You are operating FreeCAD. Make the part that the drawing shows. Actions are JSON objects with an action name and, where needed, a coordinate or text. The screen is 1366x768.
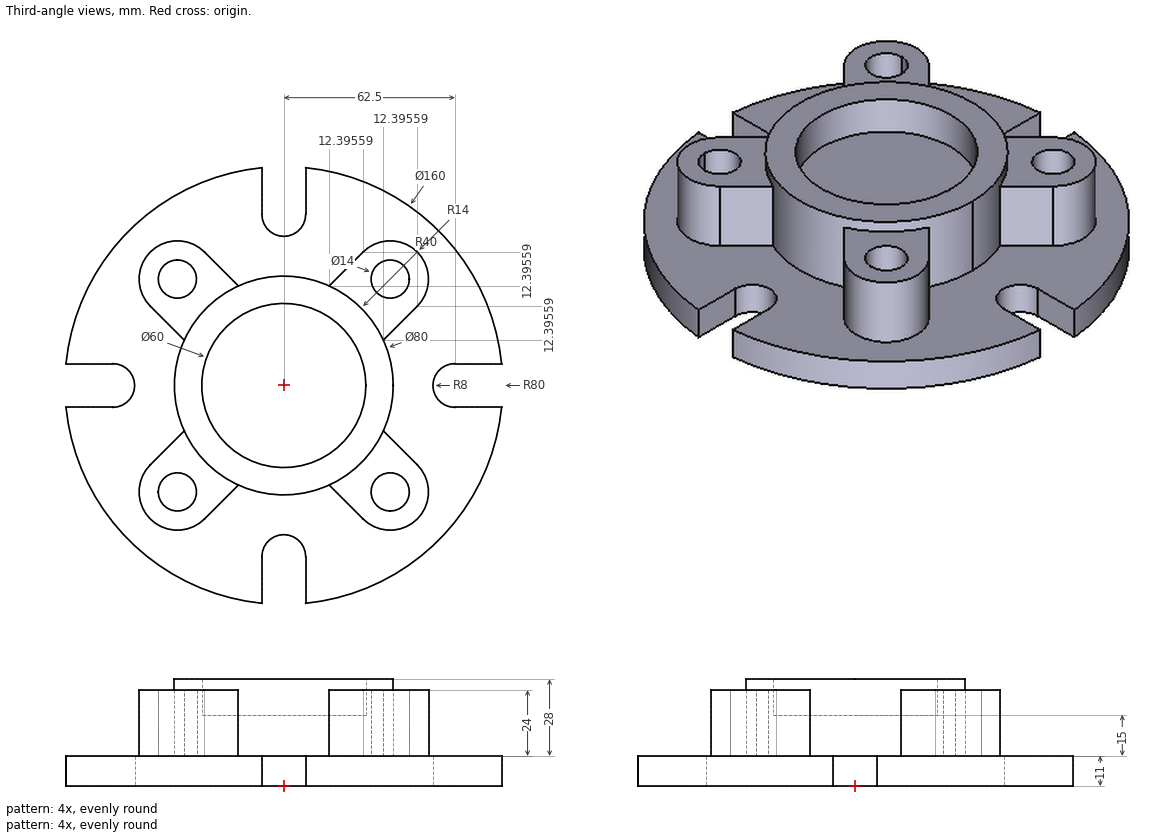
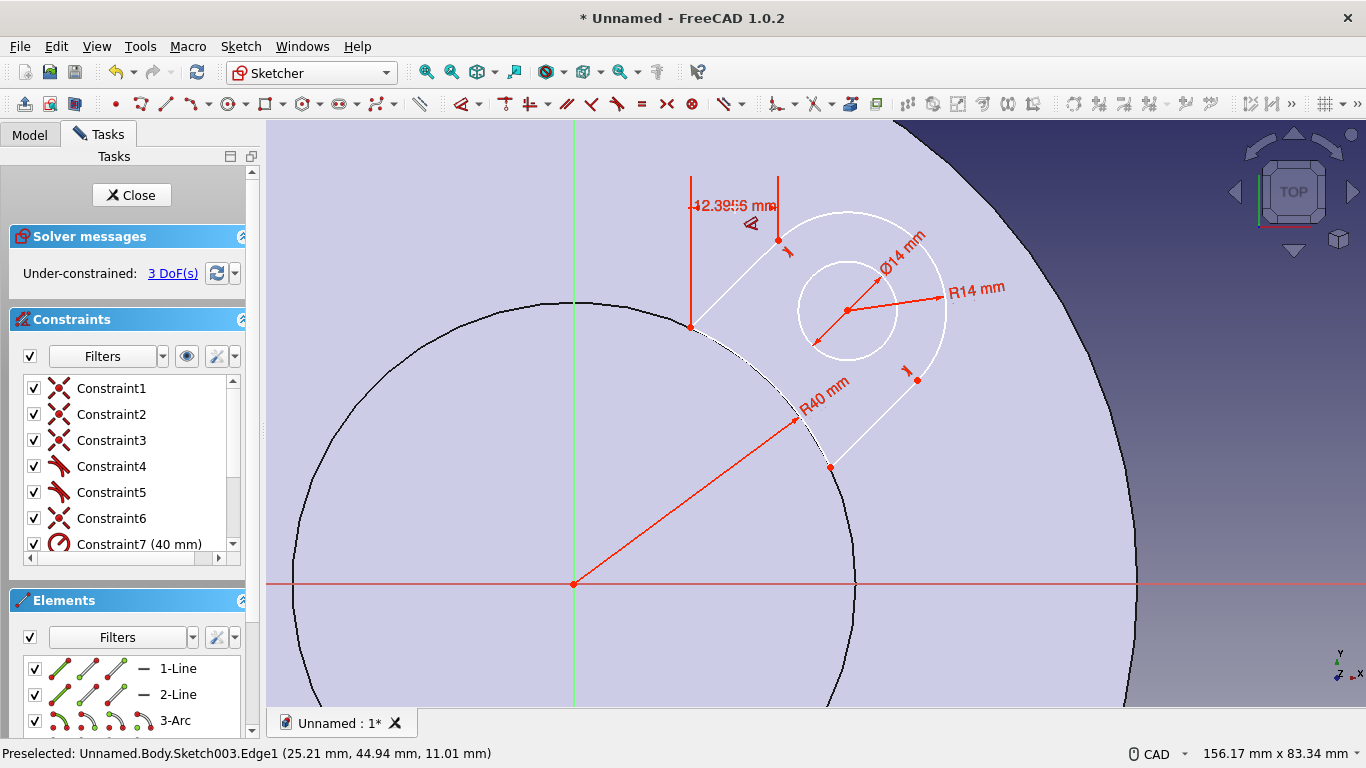
{"action": "left_click", "coordinate": [752, 267]}
{"action": "left_click", "coordinate": [657, 284]}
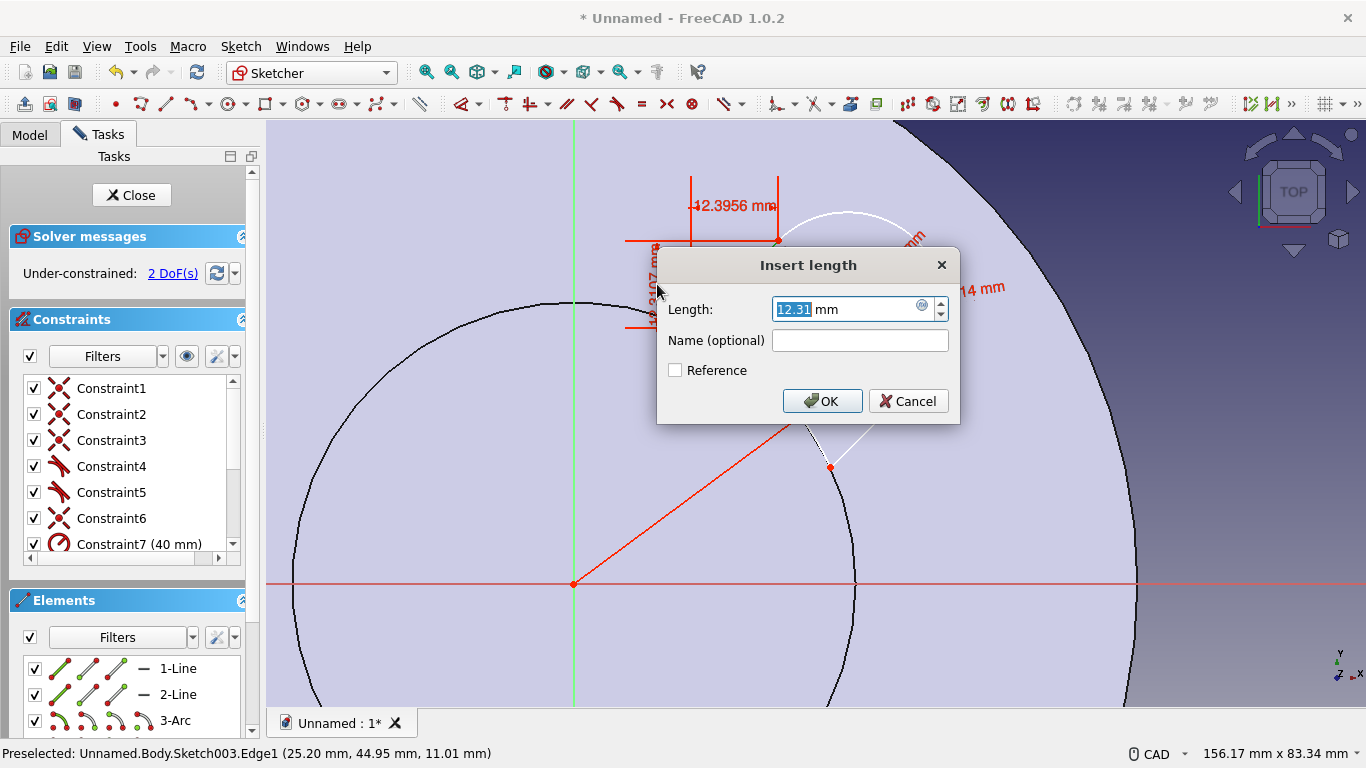
{"action": "type", "text": "12.39559"}
{"action": "key", "text": "Return"}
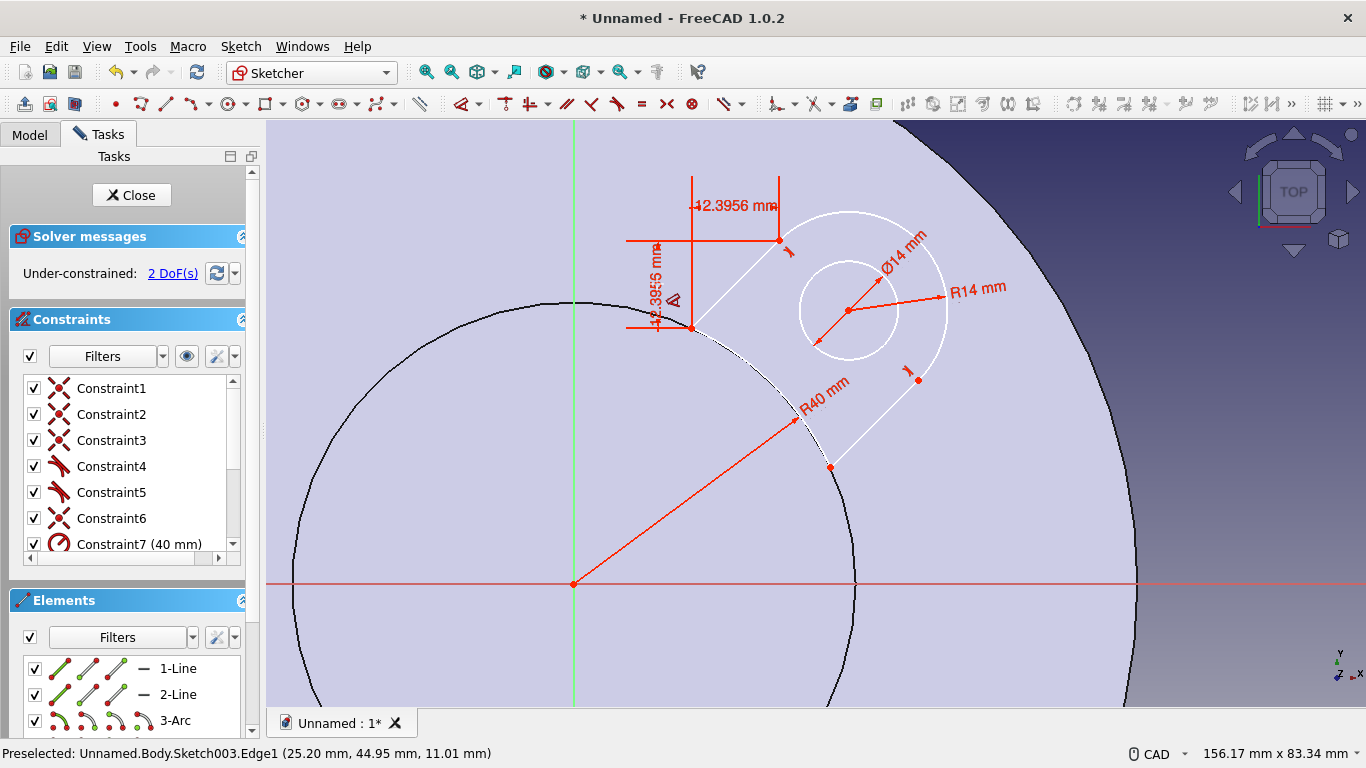
{"action": "left_click", "coordinate": [857, 442]}
{"action": "left_click", "coordinate": [875, 502]}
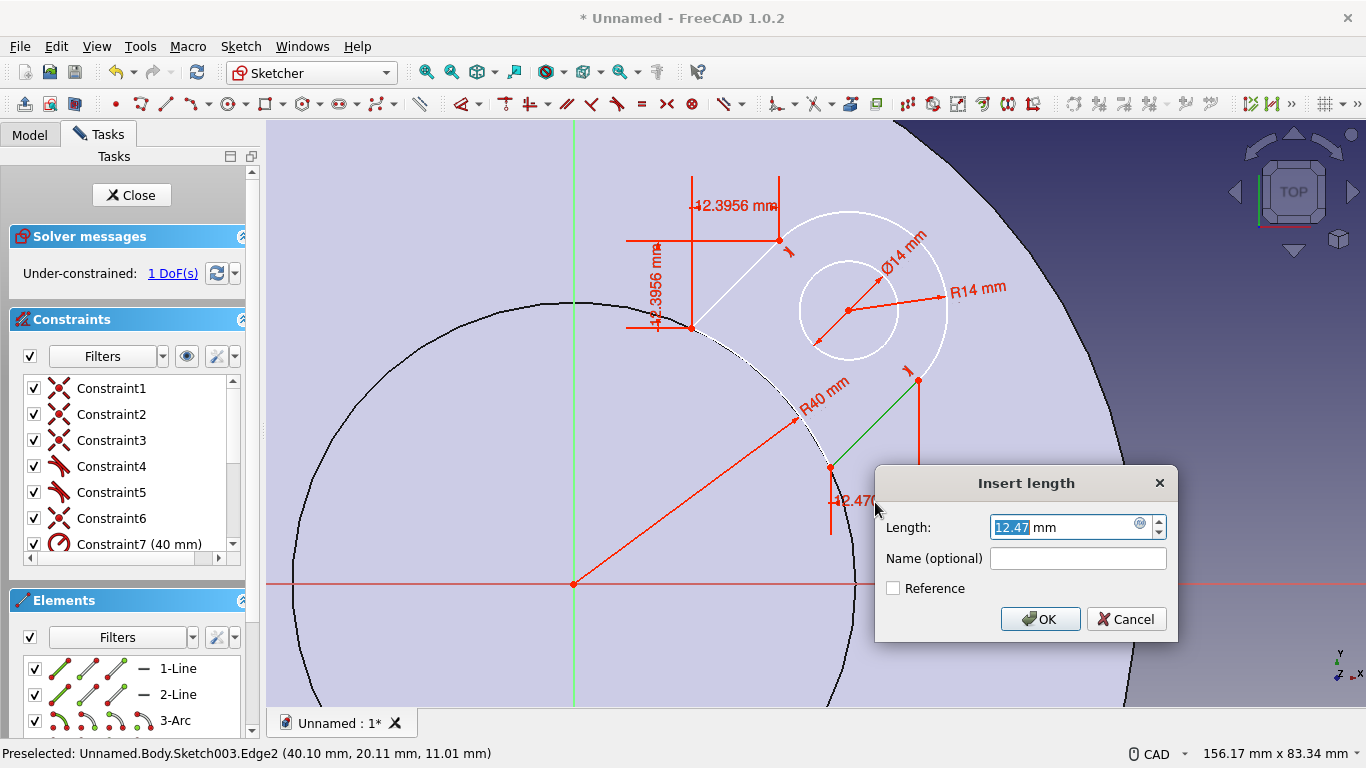
{"action": "type", "text": "12.39559"}
{"action": "key", "text": "Return"}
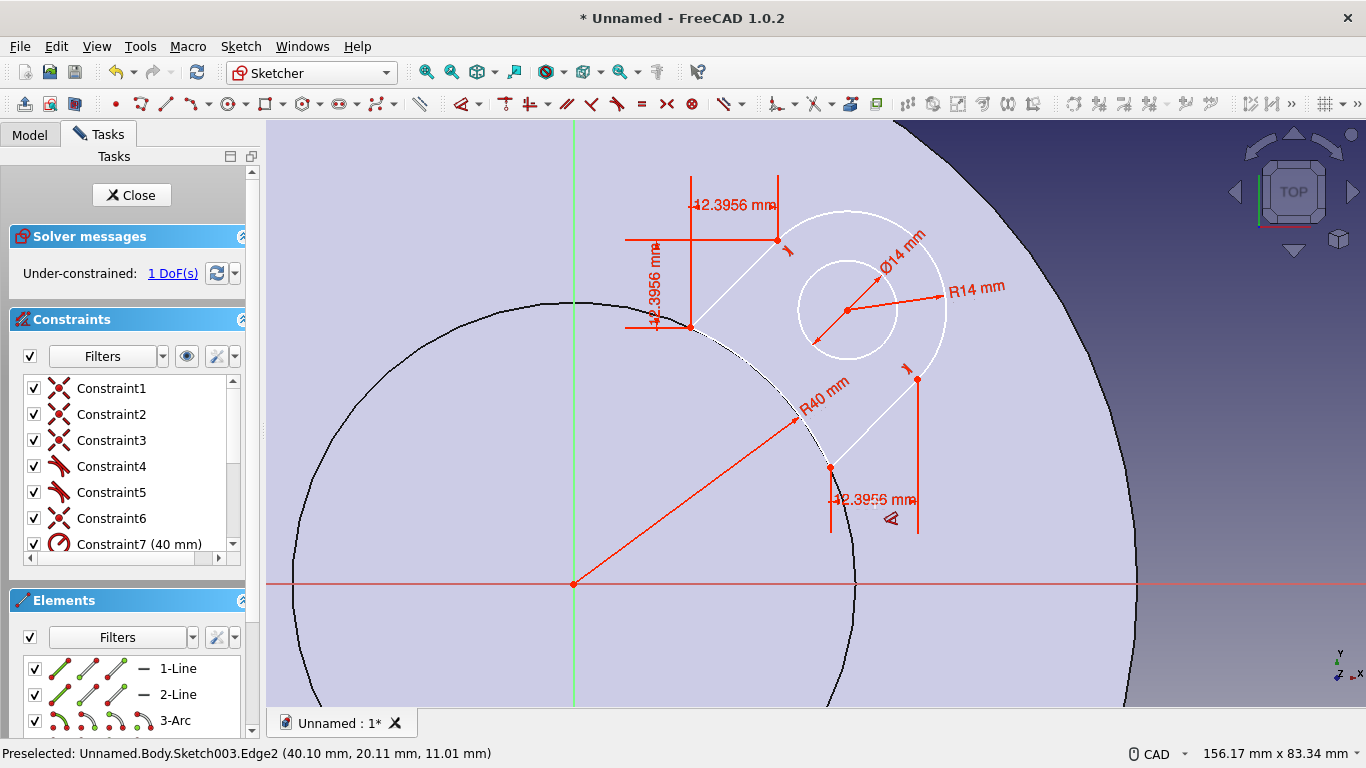
{"action": "left_click", "coordinate": [857, 441]}
{"action": "left_click", "coordinate": [952, 424]}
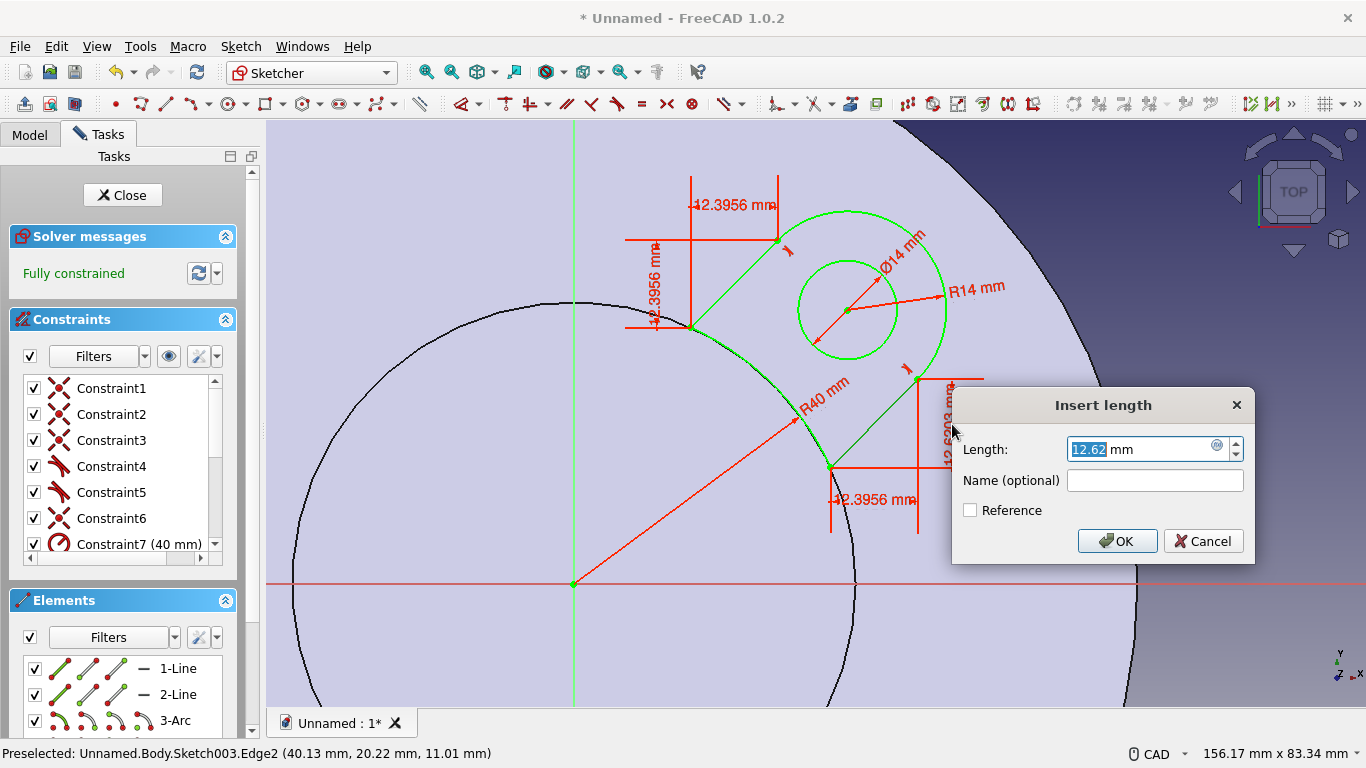
{"action": "type", "text": "12.39559"}
{"action": "key", "text": "Return"}
{"action": "key", "text": "Escape"}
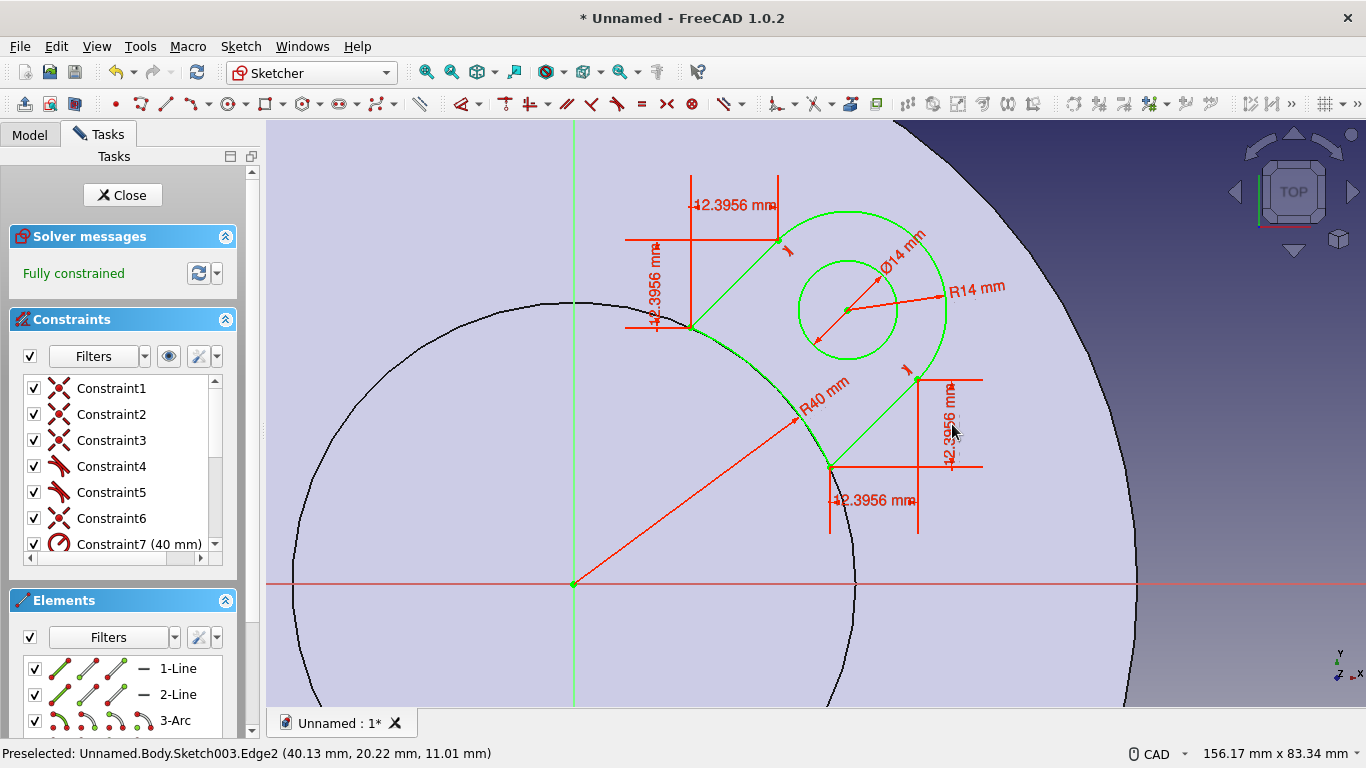
{"action": "left_click", "coordinate": [123, 195]}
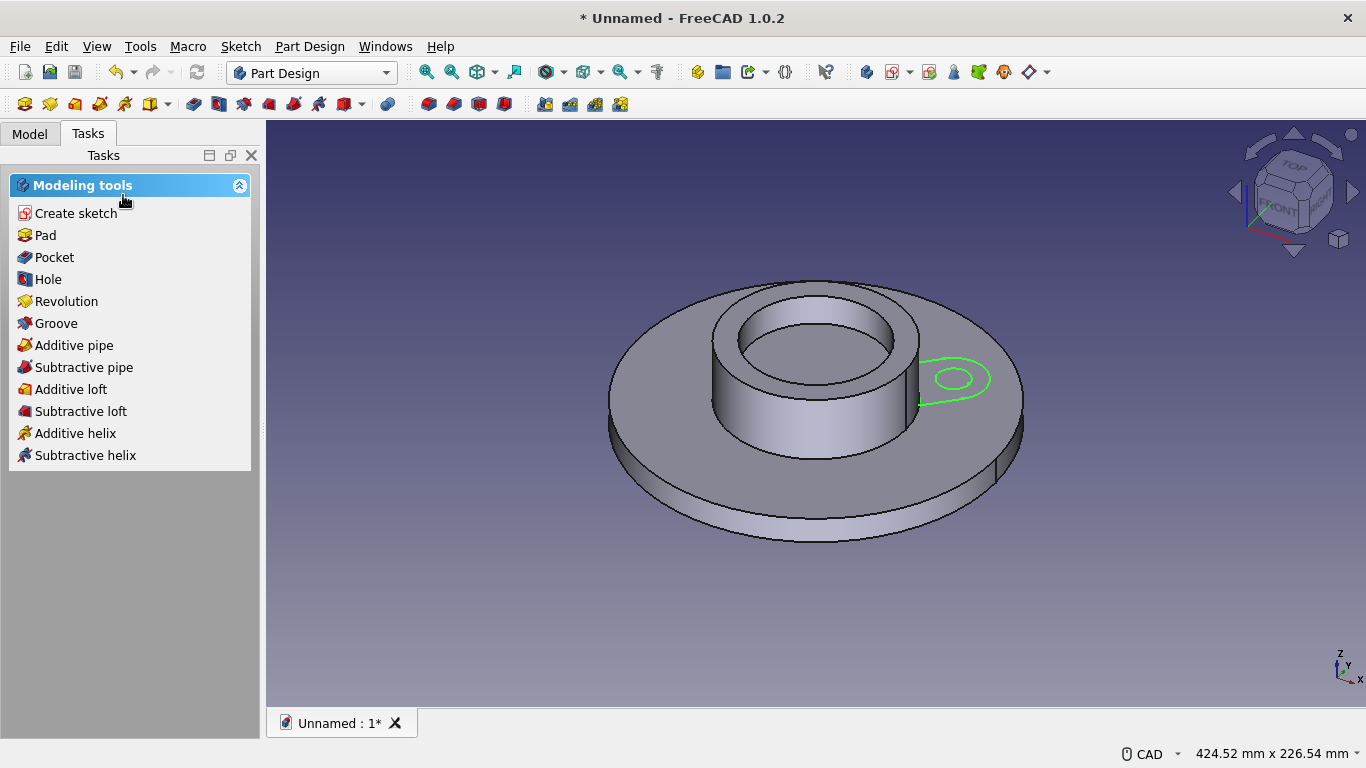
{"action": "left_click", "coordinate": [25, 104]}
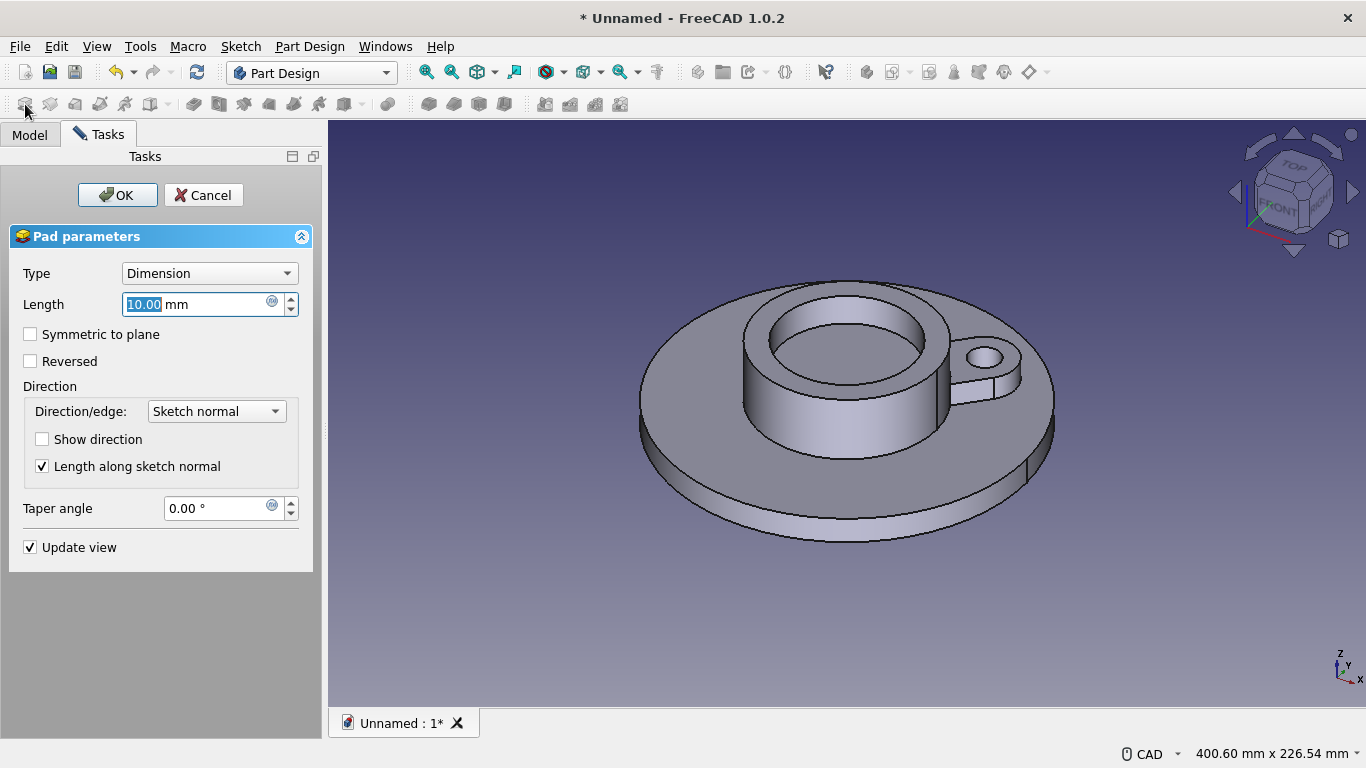
{"action": "type", "text": "24"}
{"action": "key", "text": "Tab"}